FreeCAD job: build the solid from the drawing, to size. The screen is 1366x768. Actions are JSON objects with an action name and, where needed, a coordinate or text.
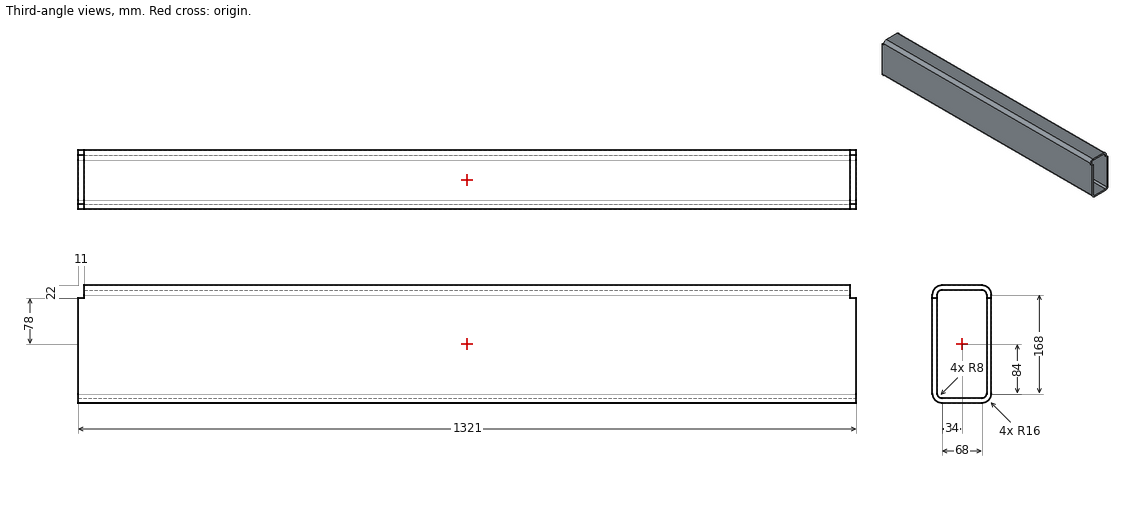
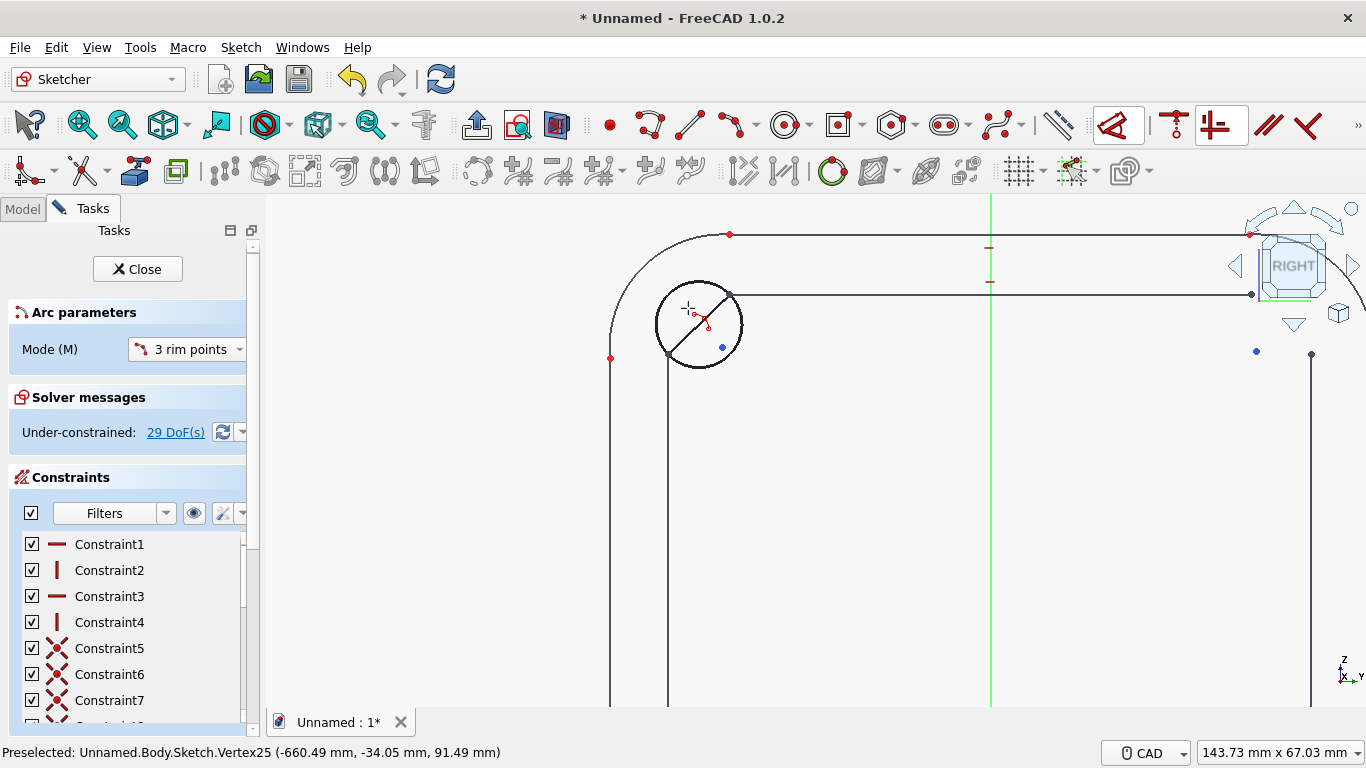
{"action": "left_click", "coordinate": [687, 309]}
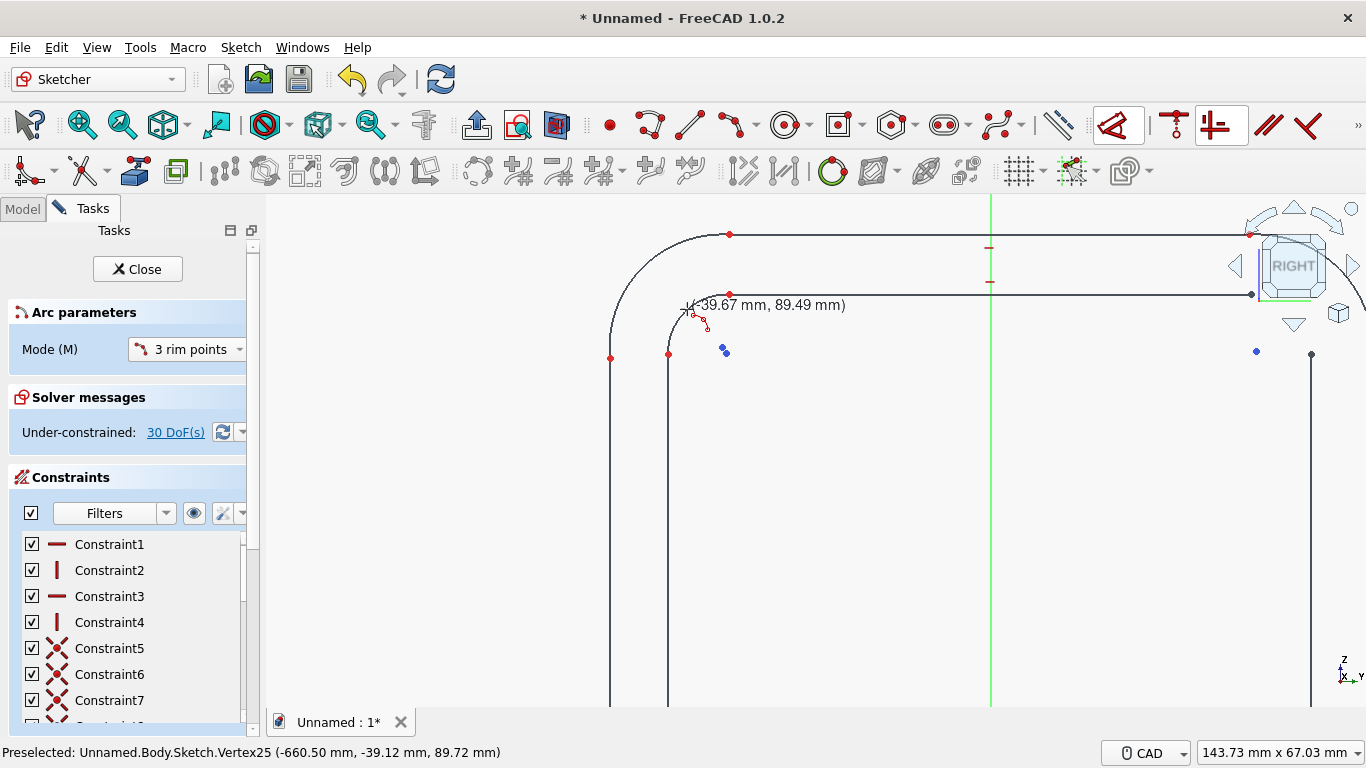
{"action": "scroll", "coordinate": [686, 313], "scroll_direction": "down", "scroll_amount": 8}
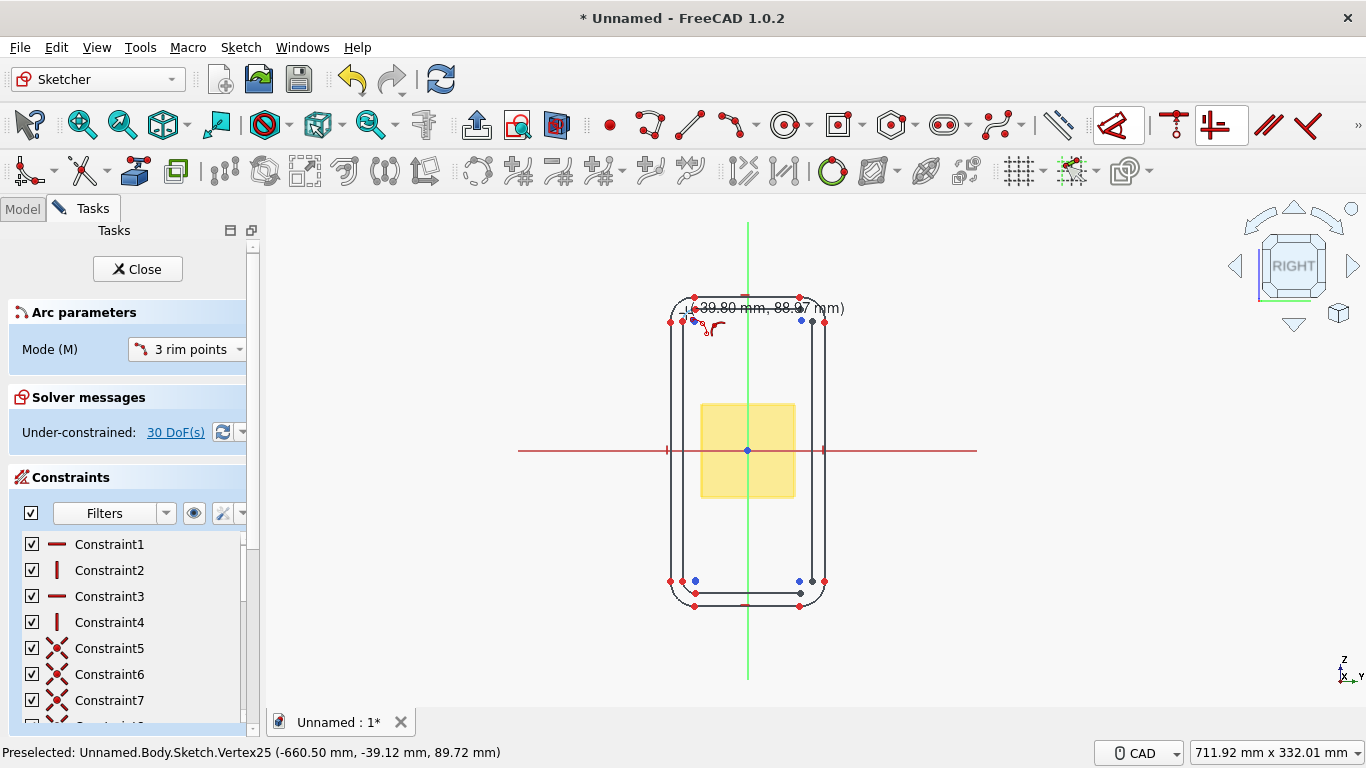
{"action": "scroll", "coordinate": [800, 309], "scroll_direction": "up", "scroll_amount": 2}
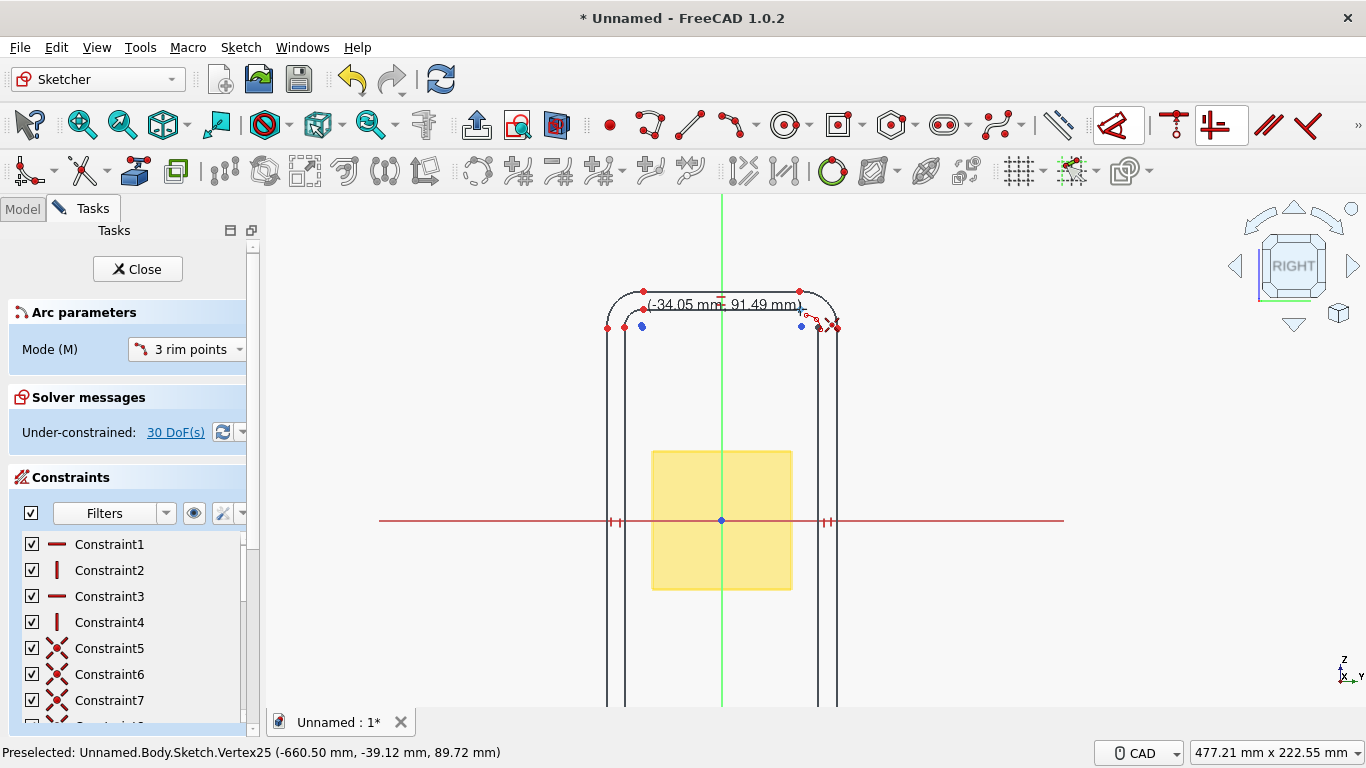
{"action": "left_click", "coordinate": [800, 310]}
{"action": "left_click", "coordinate": [818, 328]}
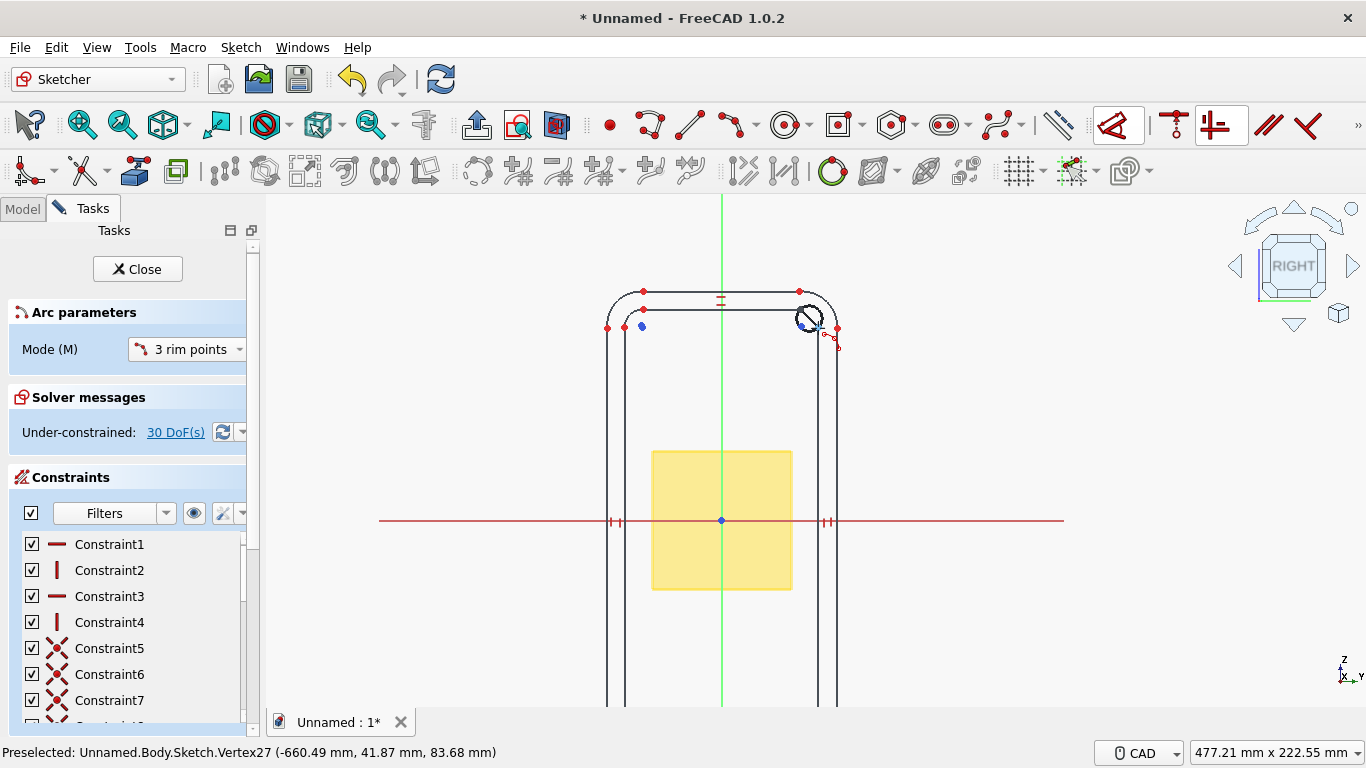
{"action": "scroll", "coordinate": [813, 314], "scroll_direction": "up", "scroll_amount": 6}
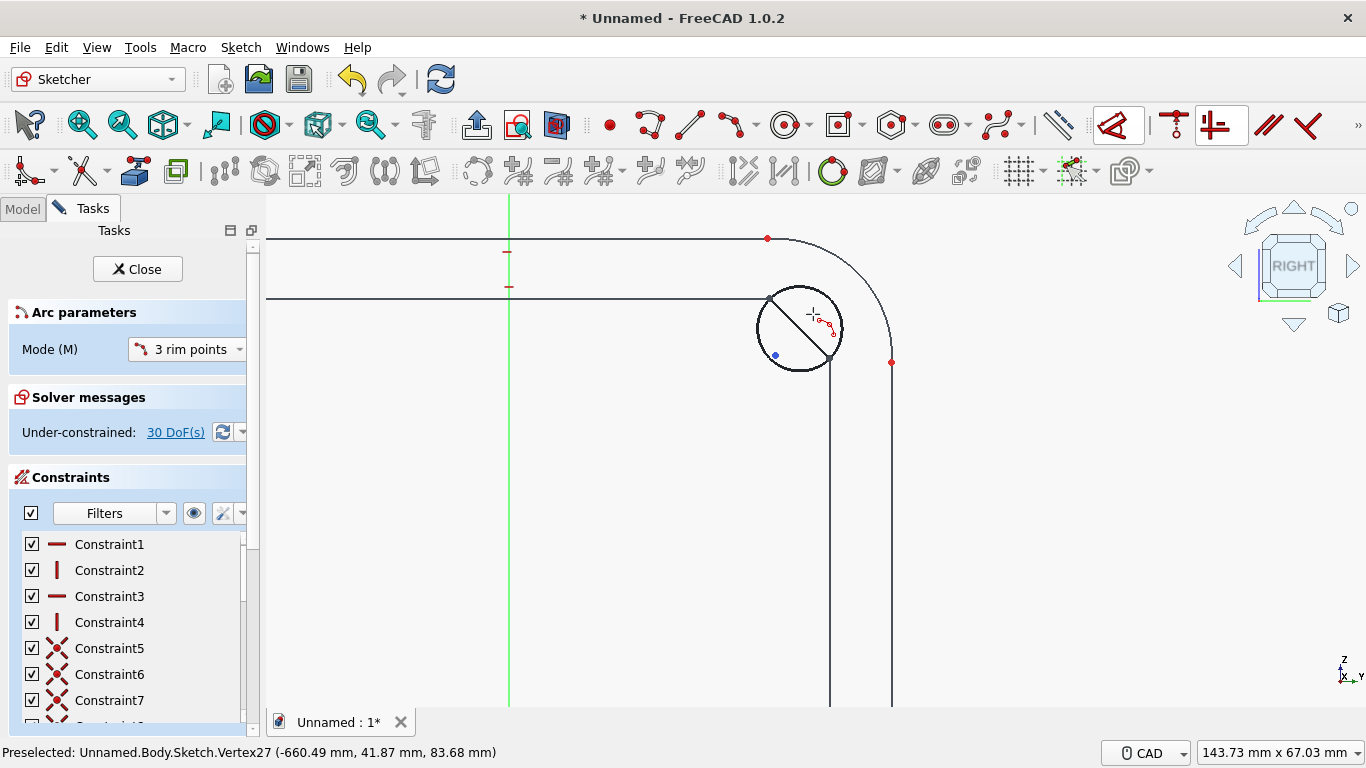
{"action": "left_click", "coordinate": [813, 313]}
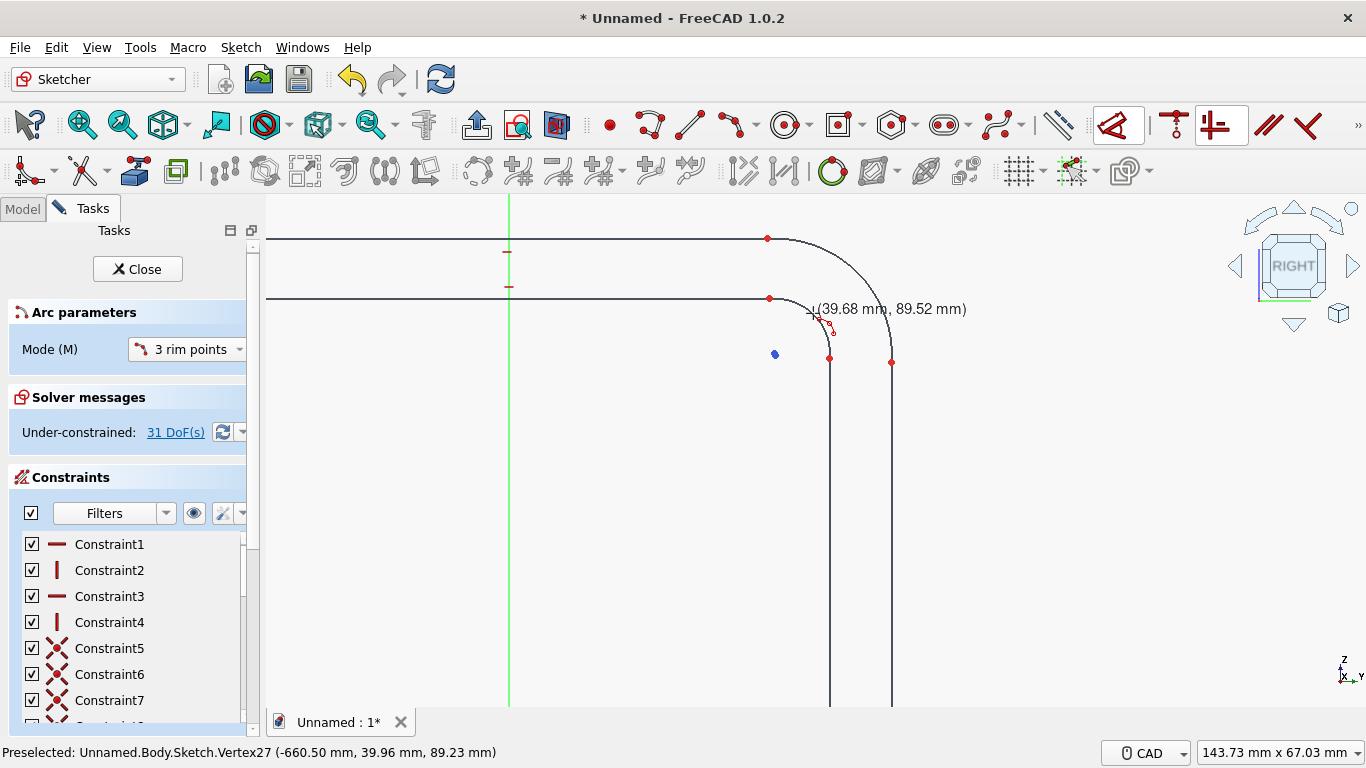
{"action": "scroll", "coordinate": [808, 312], "scroll_direction": "down", "scroll_amount": 8}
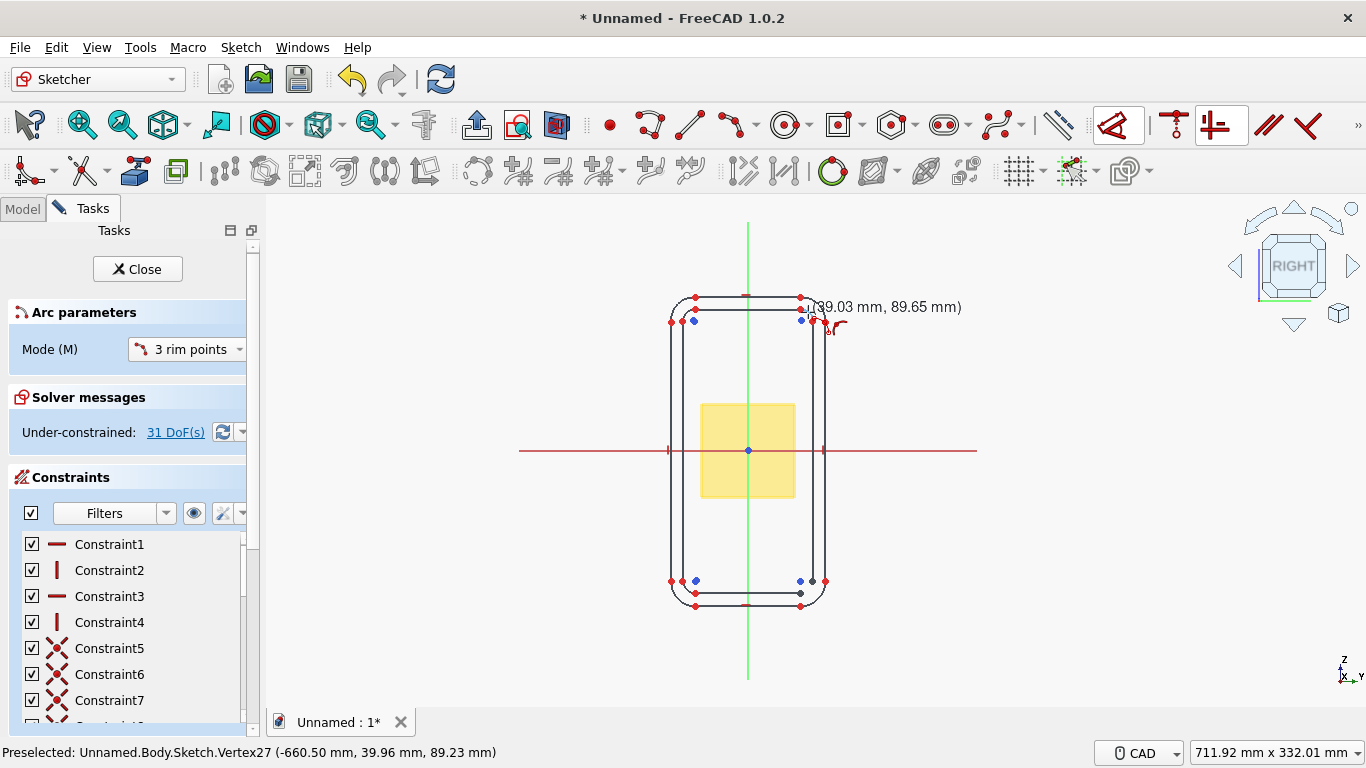
{"action": "scroll", "coordinate": [813, 581], "scroll_direction": "up", "scroll_amount": 2}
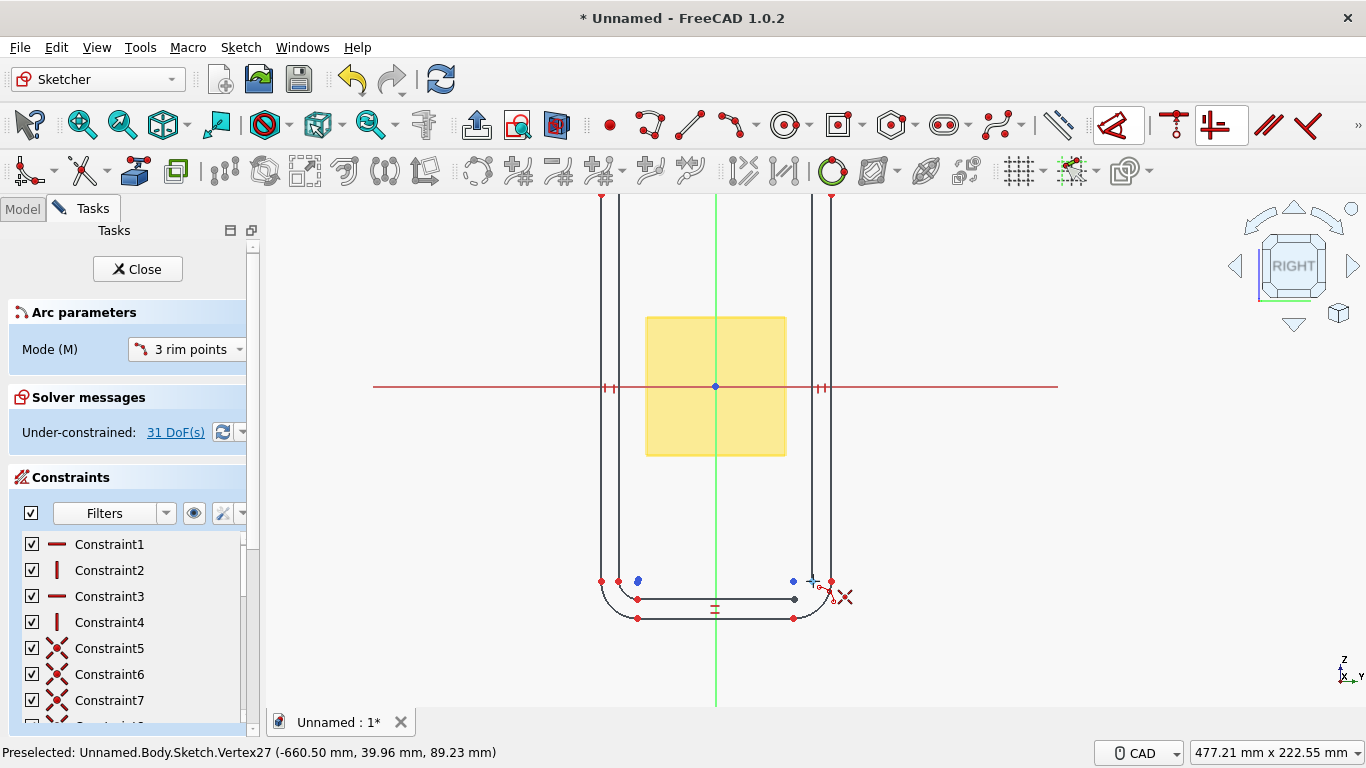
{"action": "left_click", "coordinate": [812, 581]}
{"action": "left_click", "coordinate": [794, 599]}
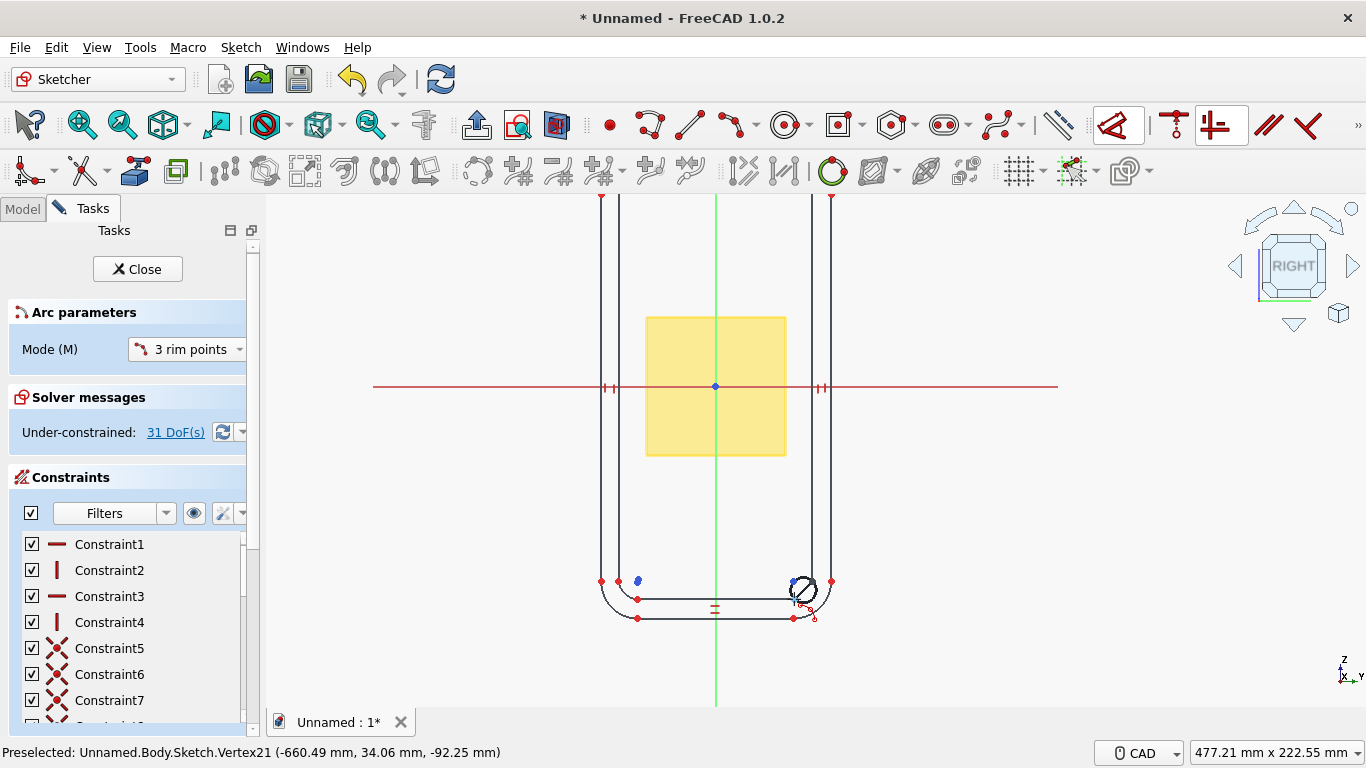
{"action": "scroll", "coordinate": [807, 593], "scroll_direction": "up", "scroll_amount": 6}